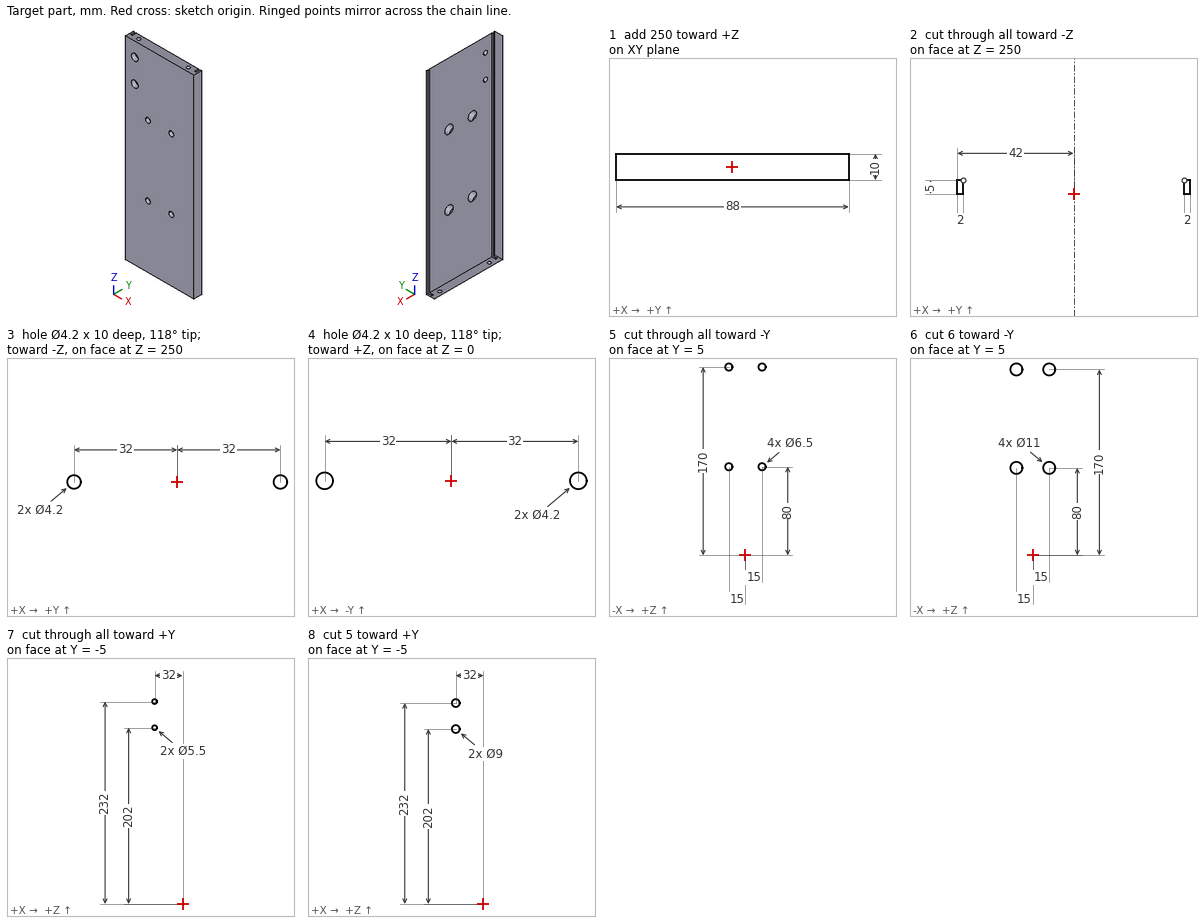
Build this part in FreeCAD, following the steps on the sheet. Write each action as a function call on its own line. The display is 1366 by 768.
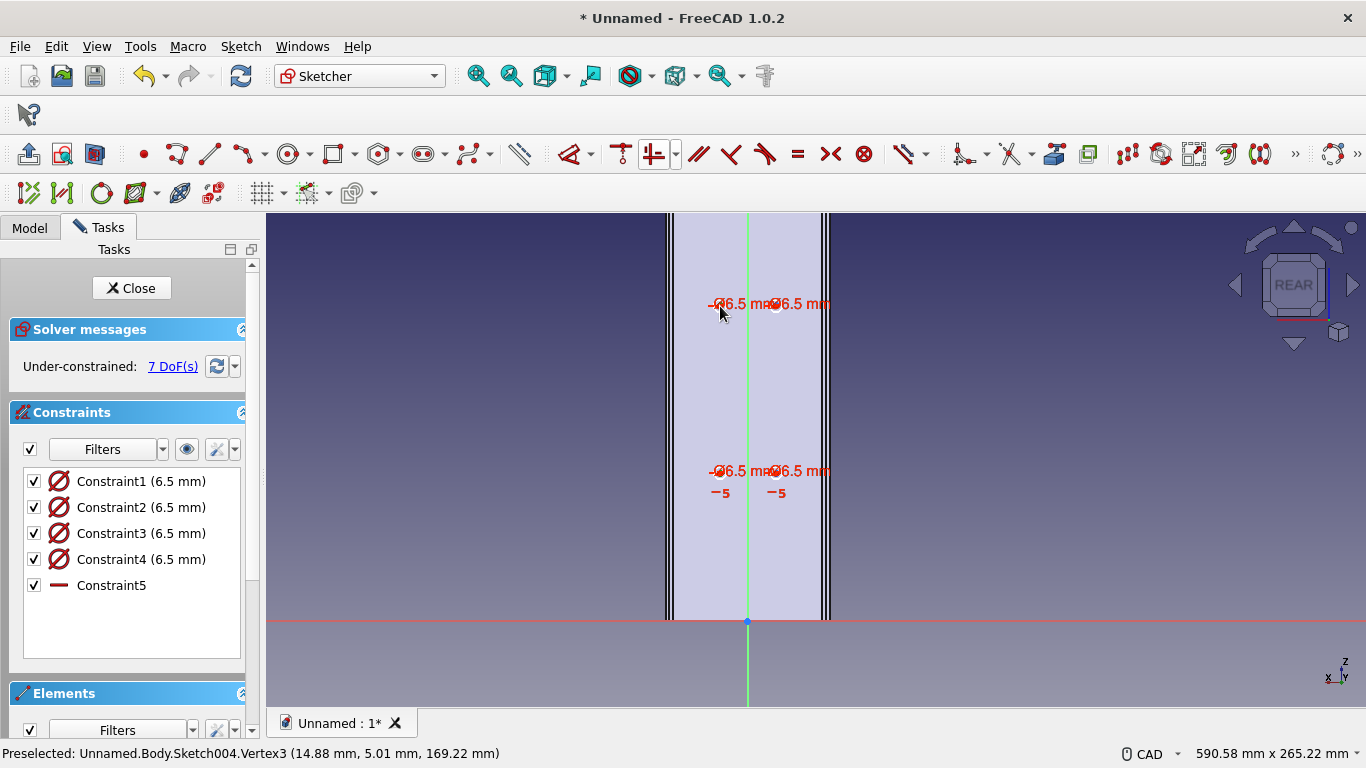
click(676, 154)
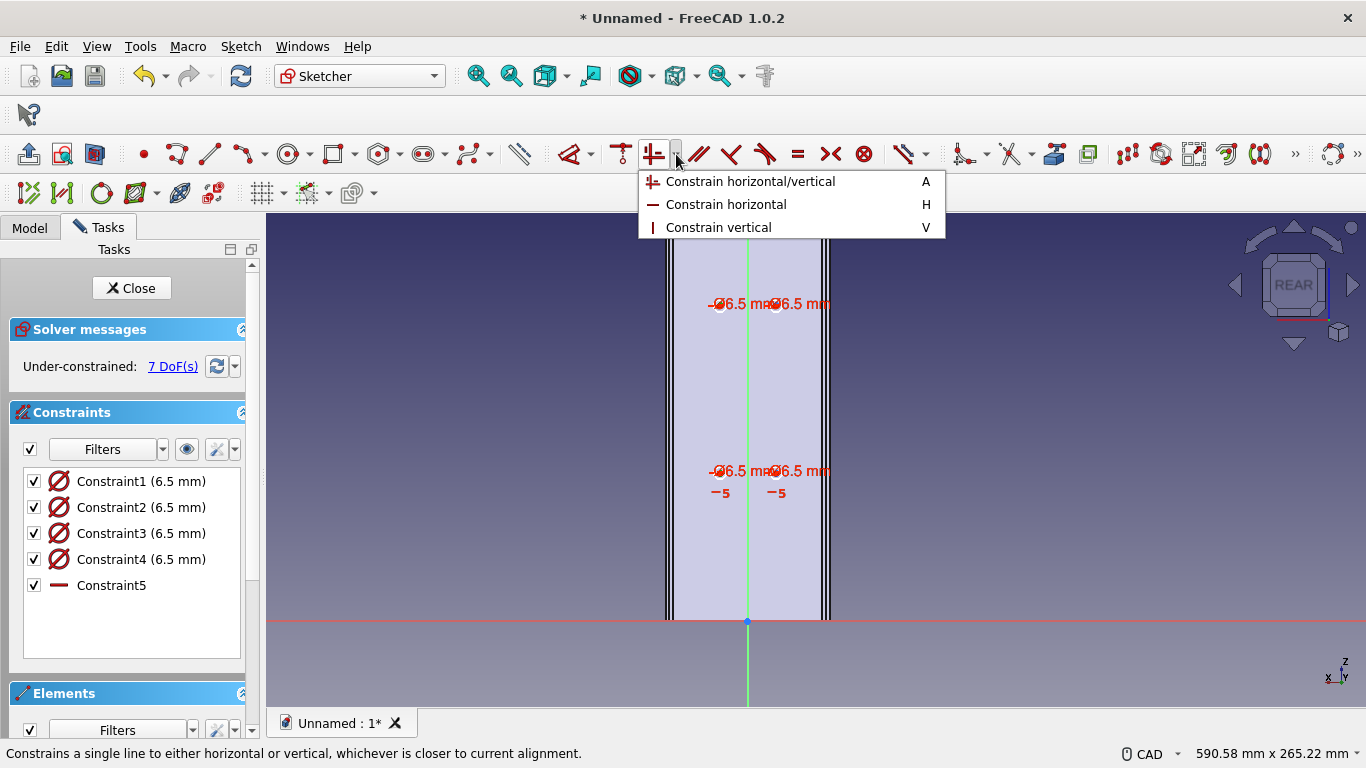
click(792, 228)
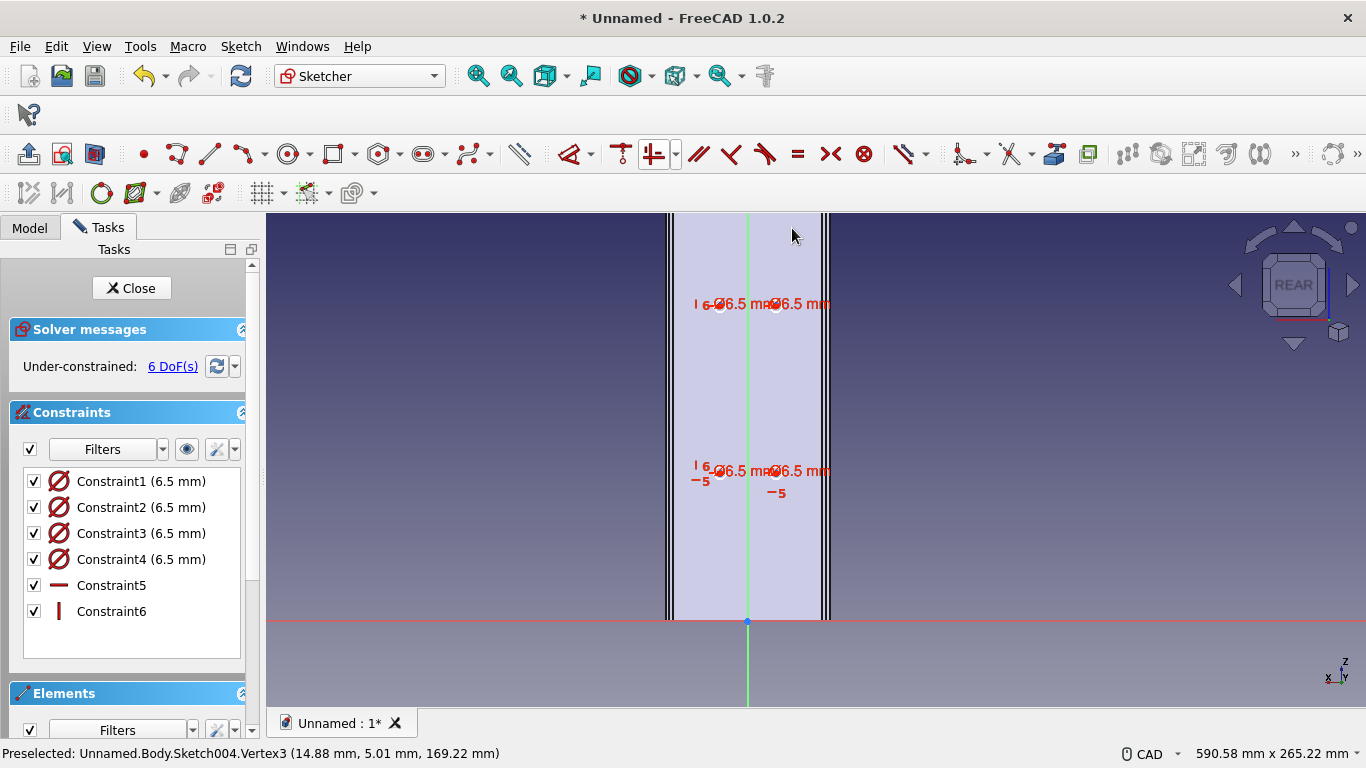
click(776, 473)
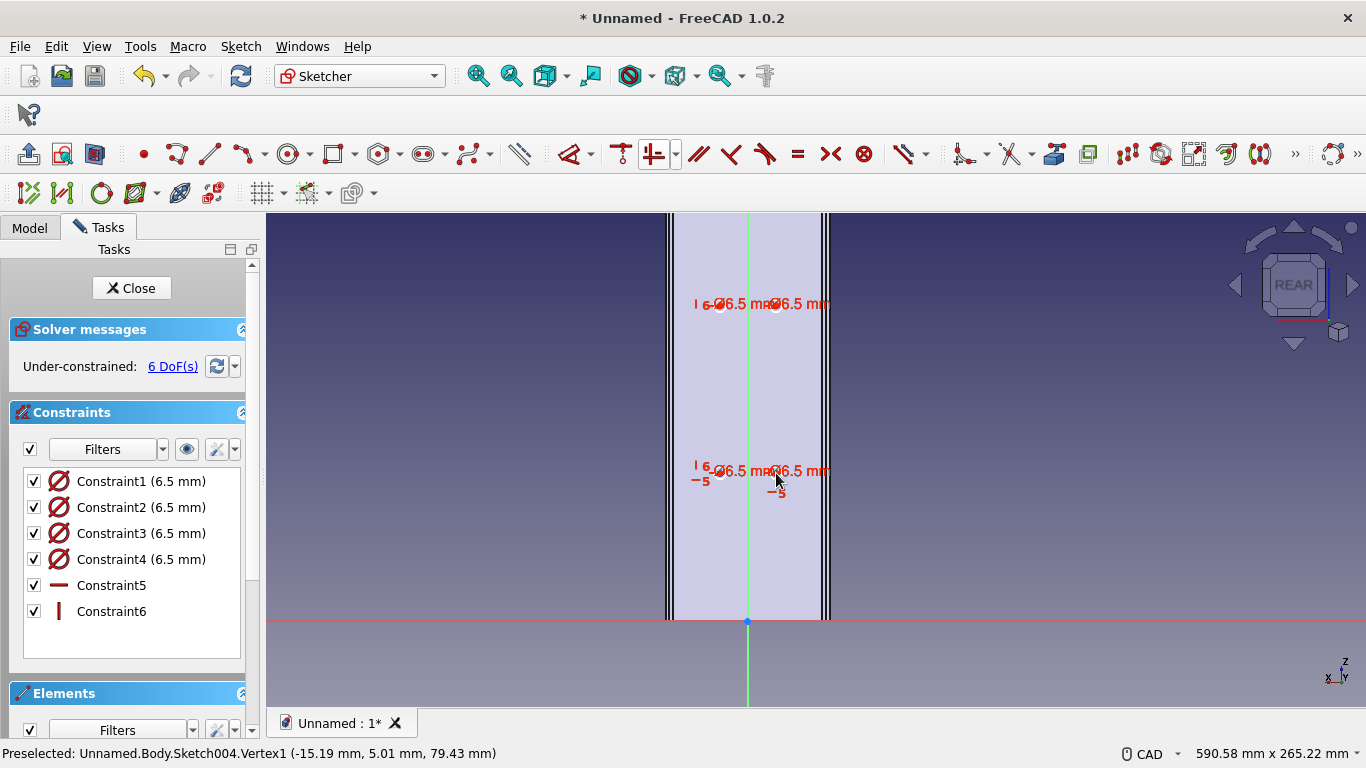
click(776, 306)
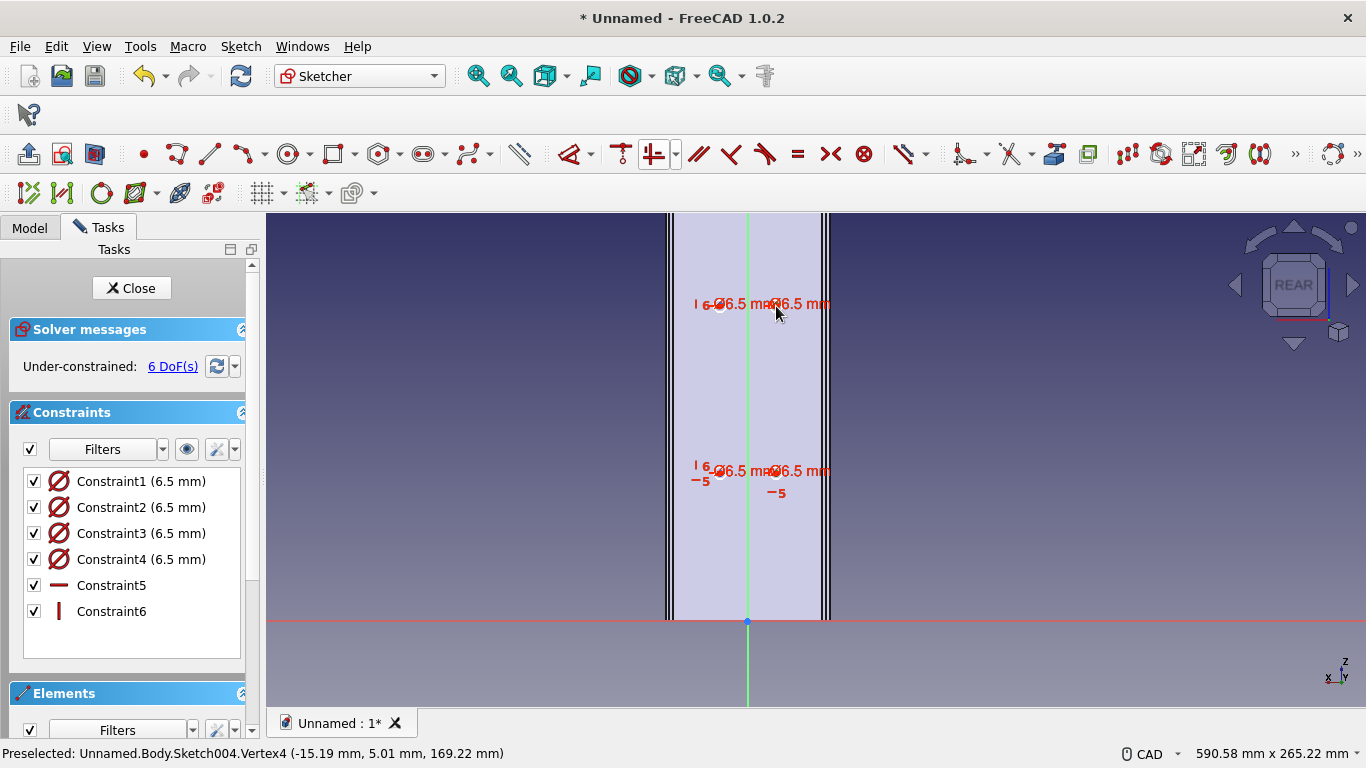
click(676, 154)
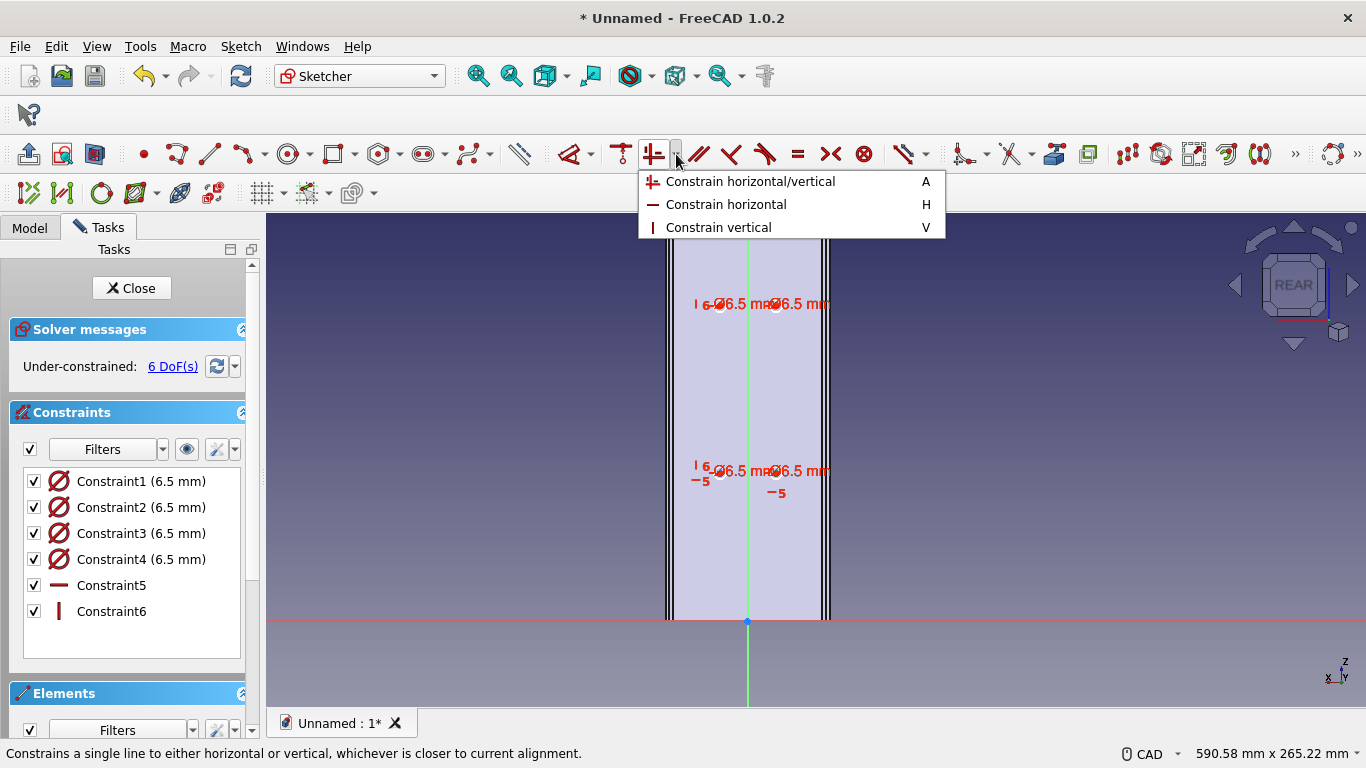
click(792, 228)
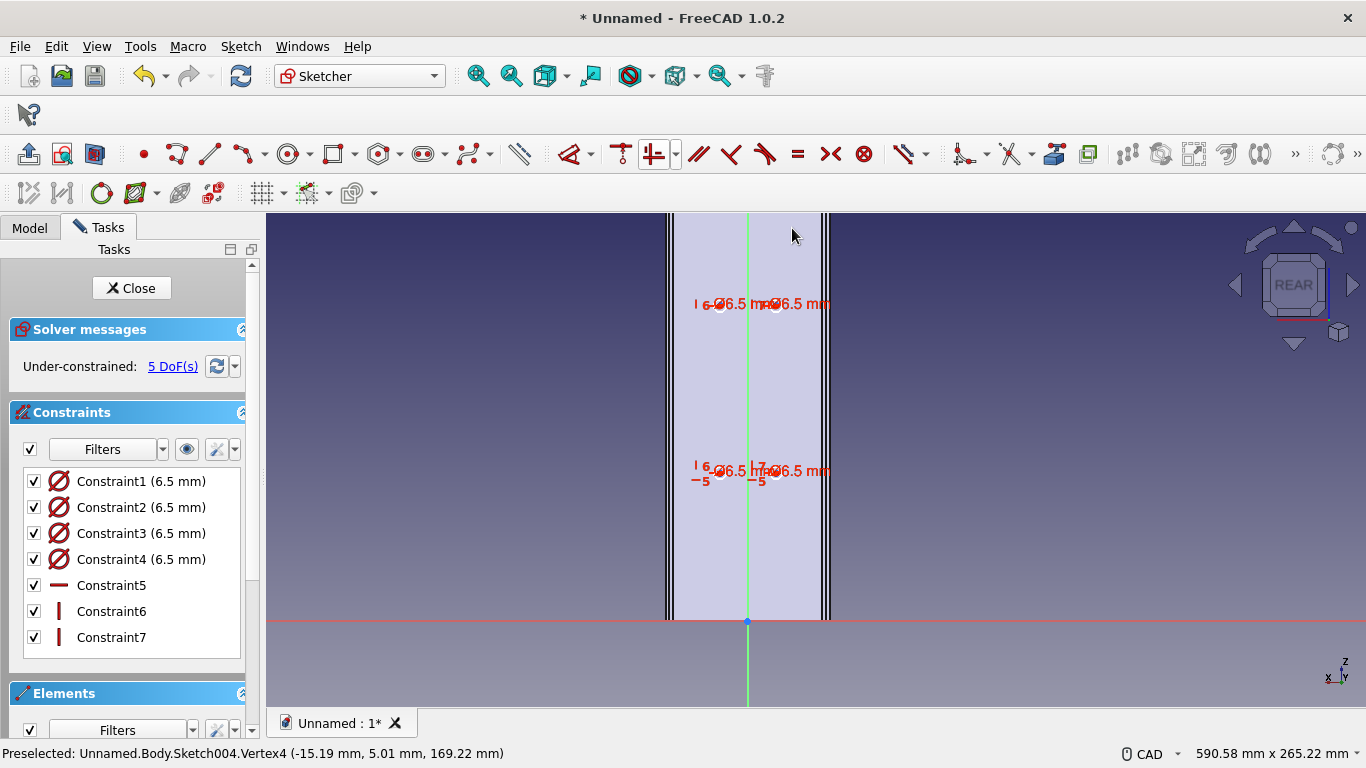
click(720, 306)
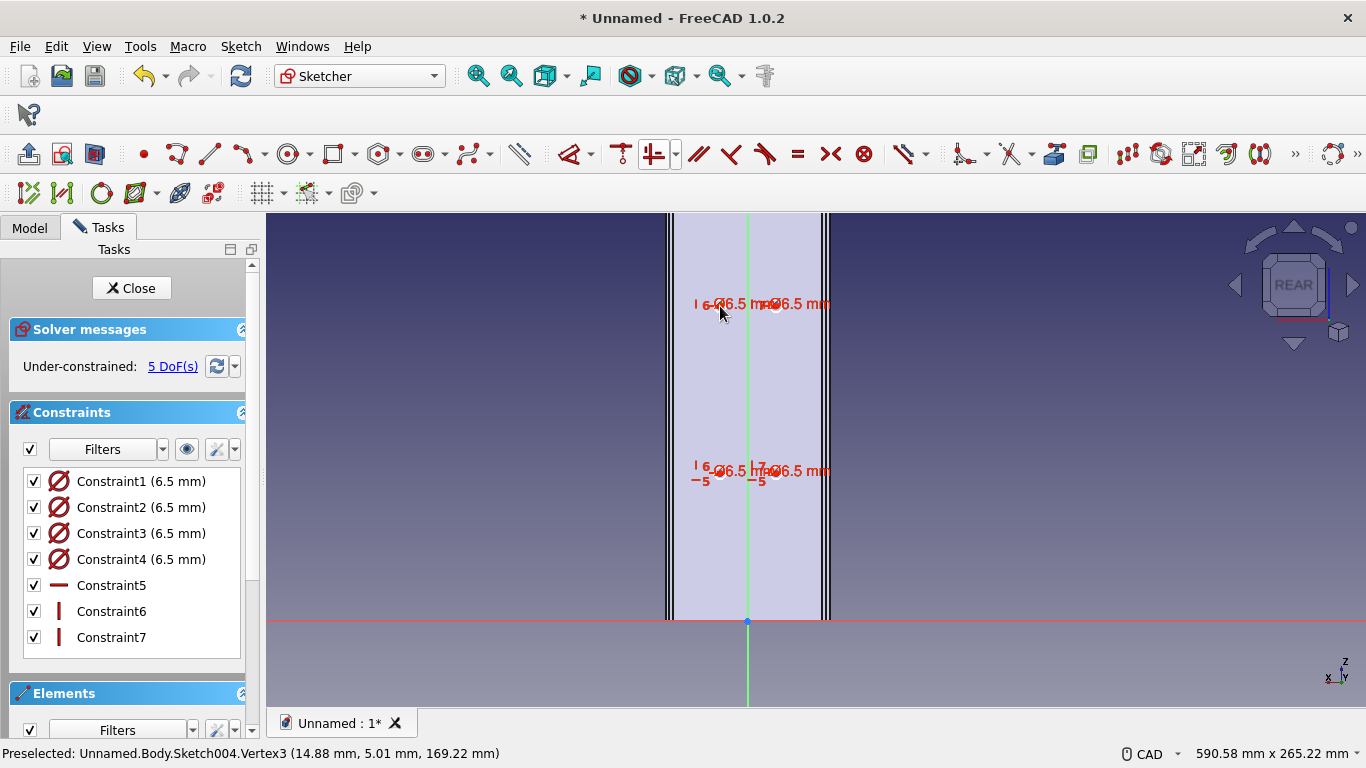
click(776, 306)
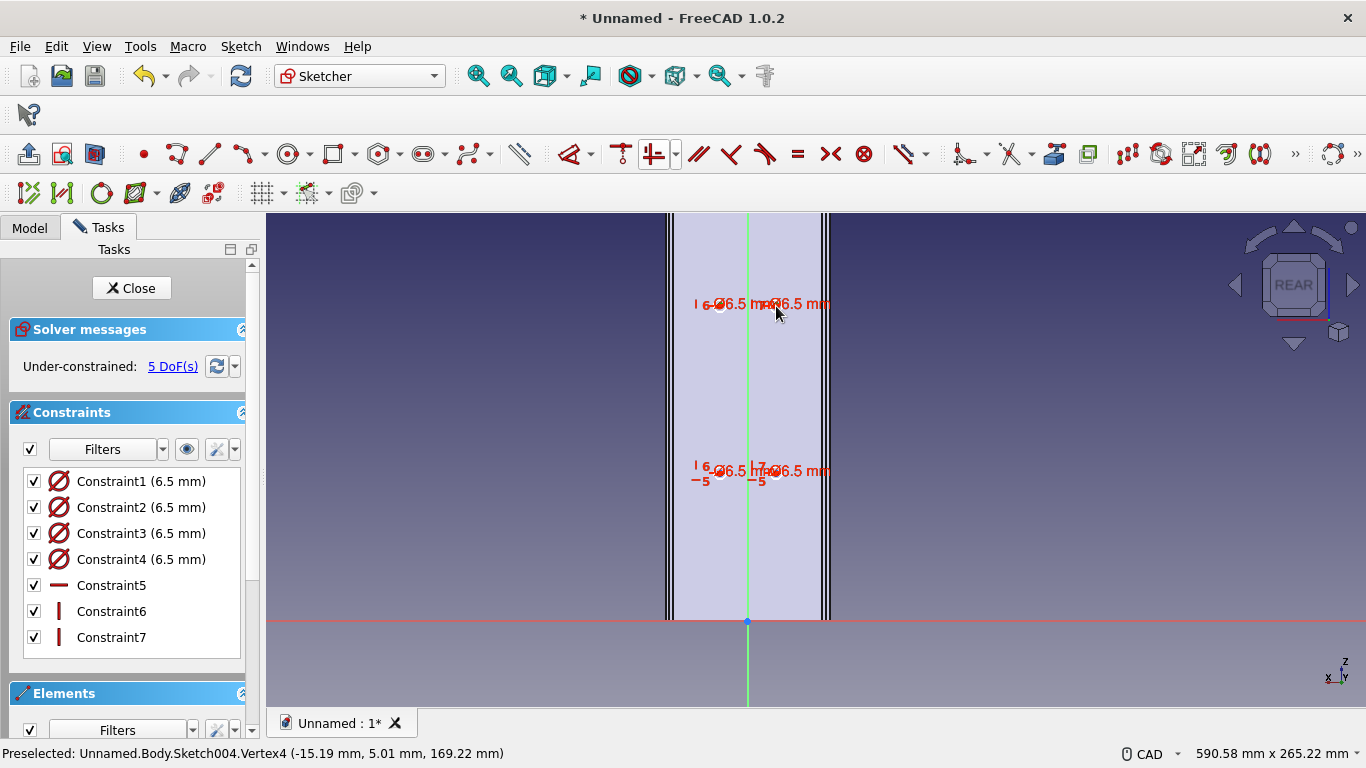
click(676, 154)